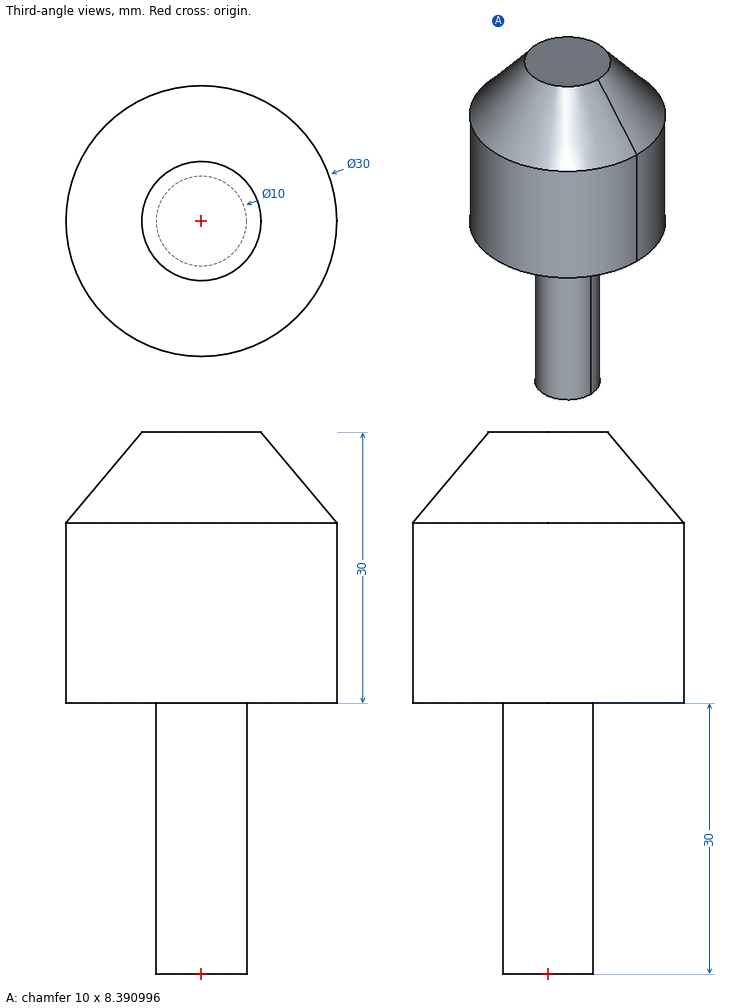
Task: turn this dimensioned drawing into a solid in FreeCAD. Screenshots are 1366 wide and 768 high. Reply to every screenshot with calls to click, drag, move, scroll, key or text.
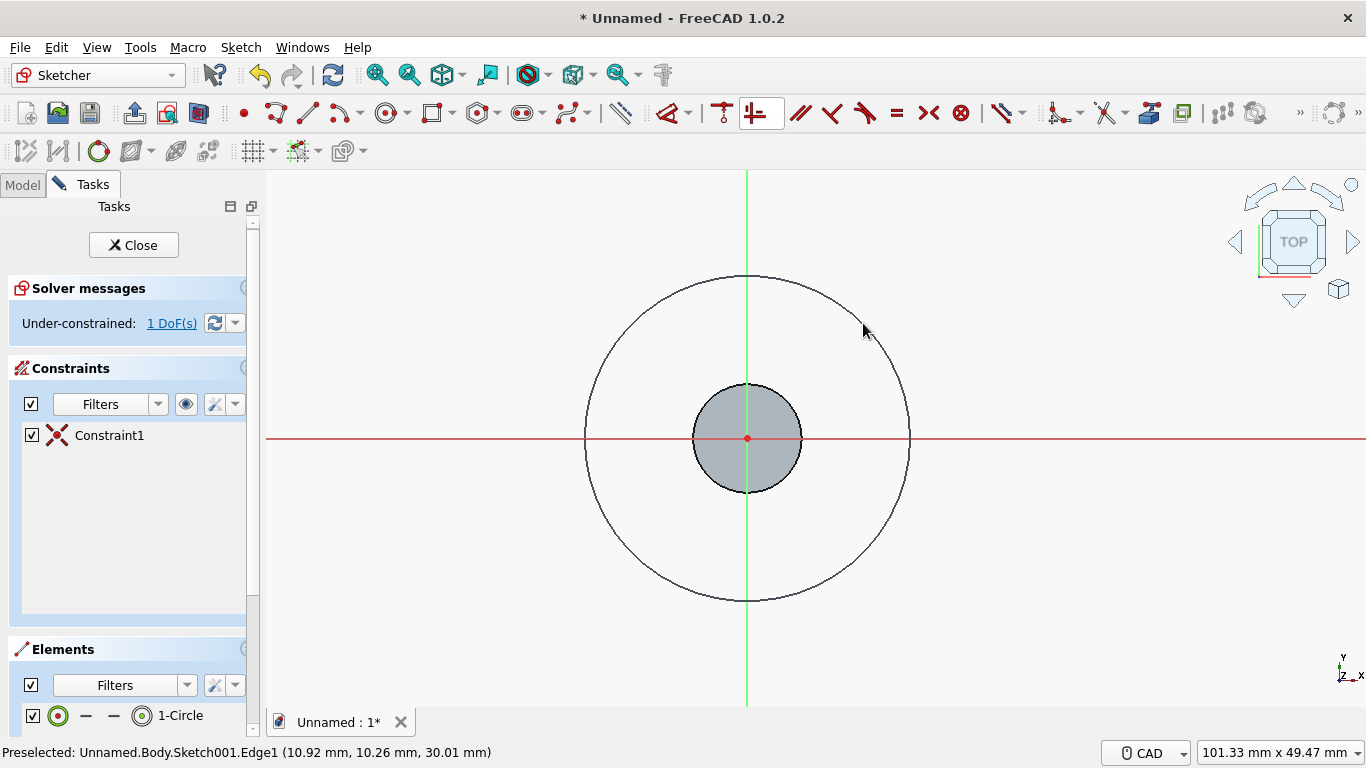
click(668, 114)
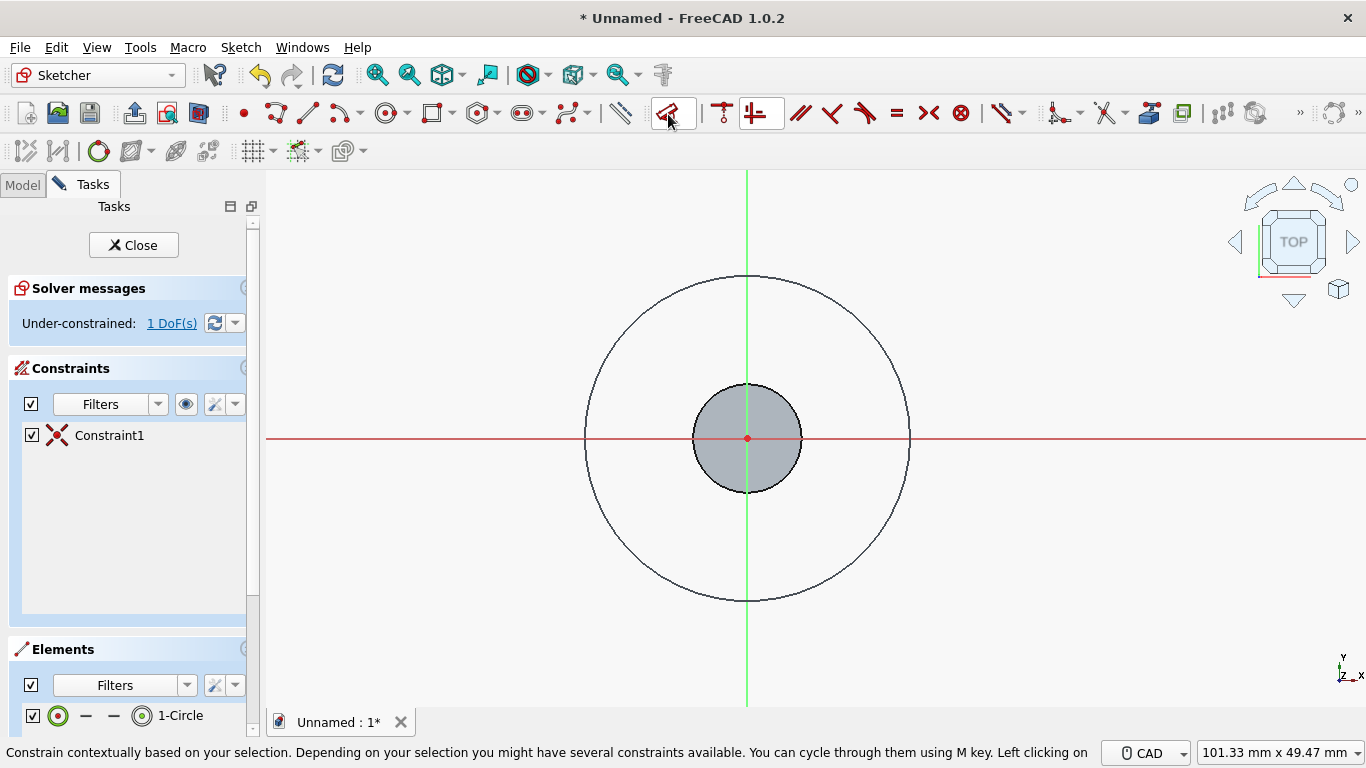
click(862, 323)
click(885, 300)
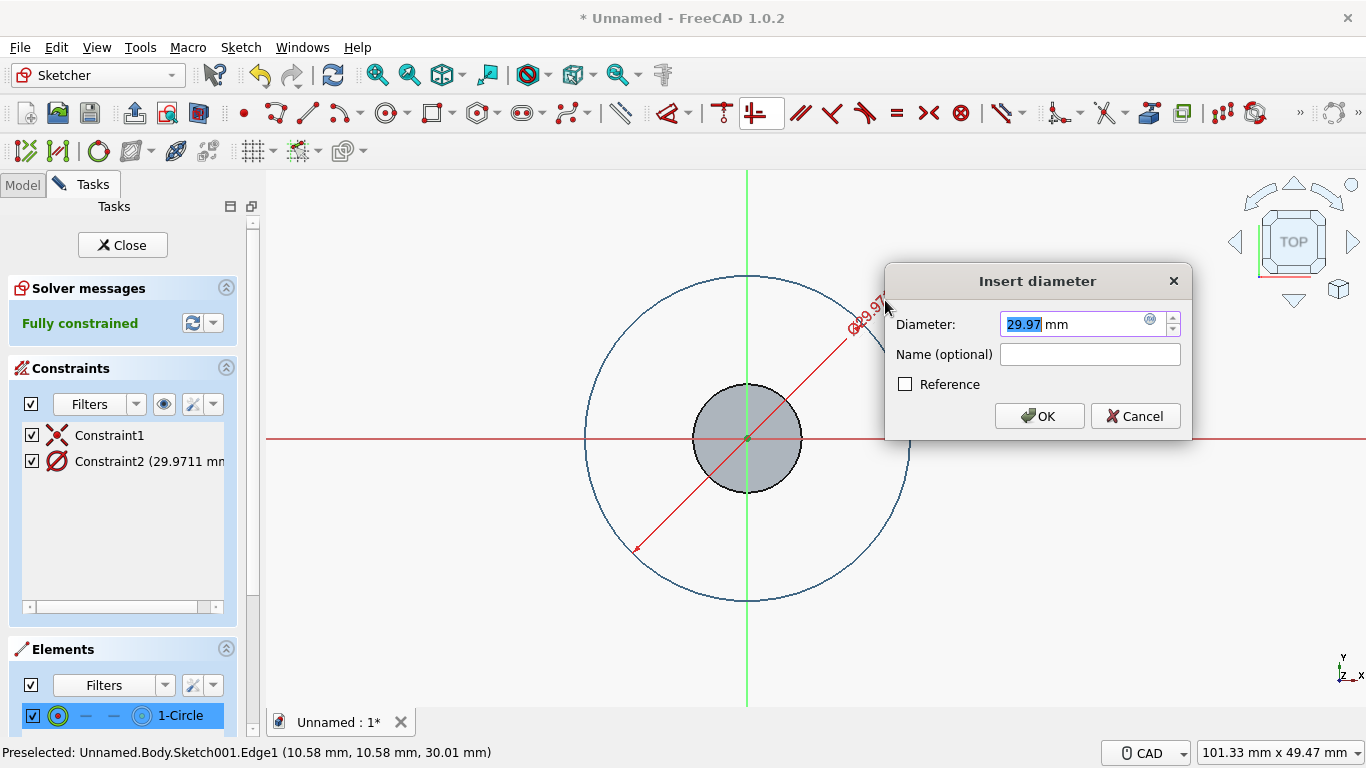
text(30)
key(Return)
key(Escape)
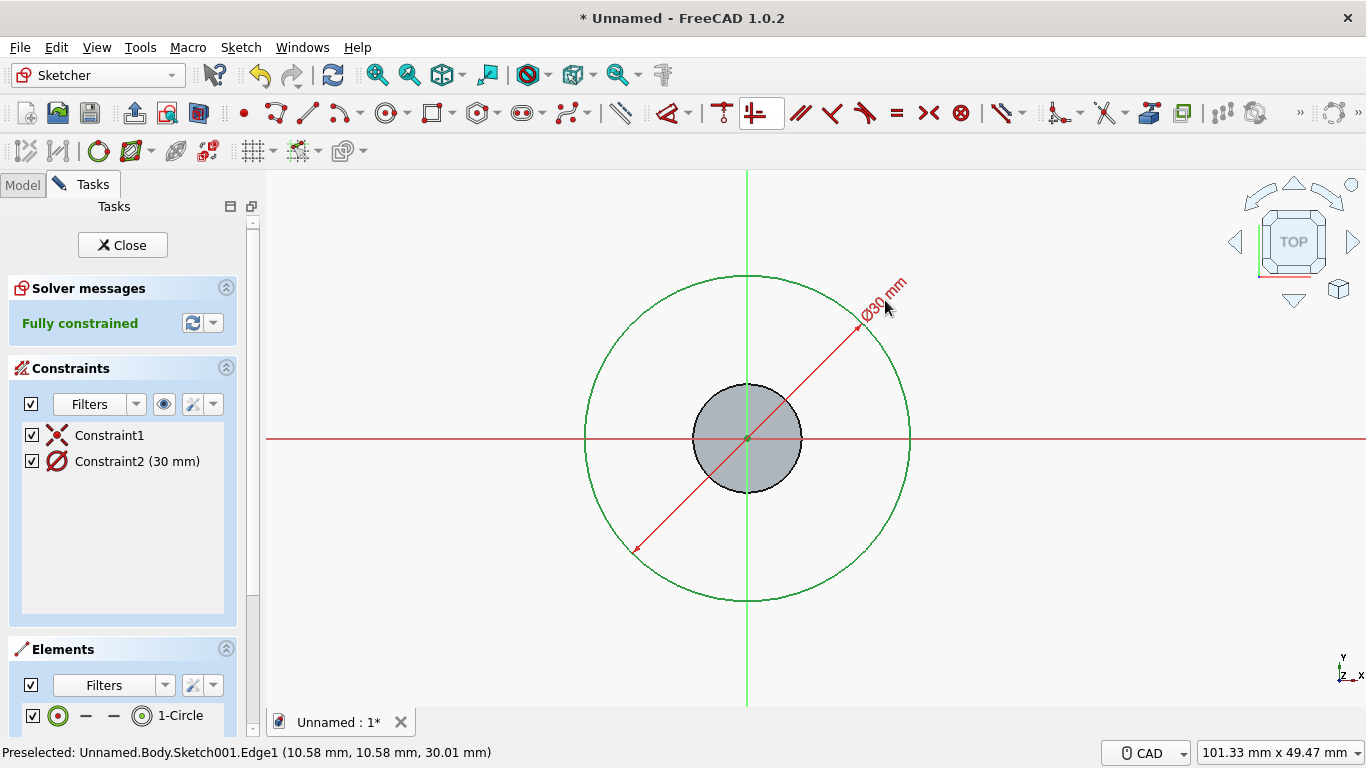
click(123, 245)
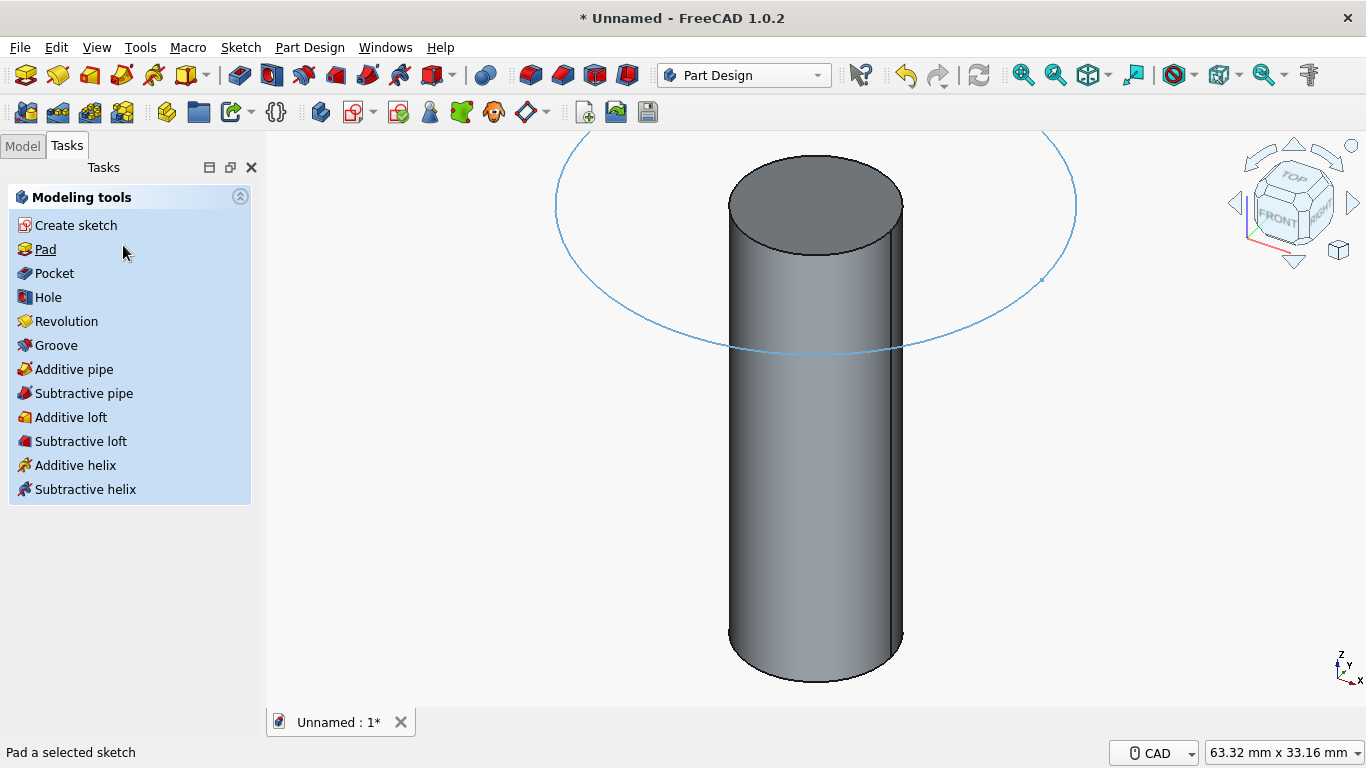
click(26, 76)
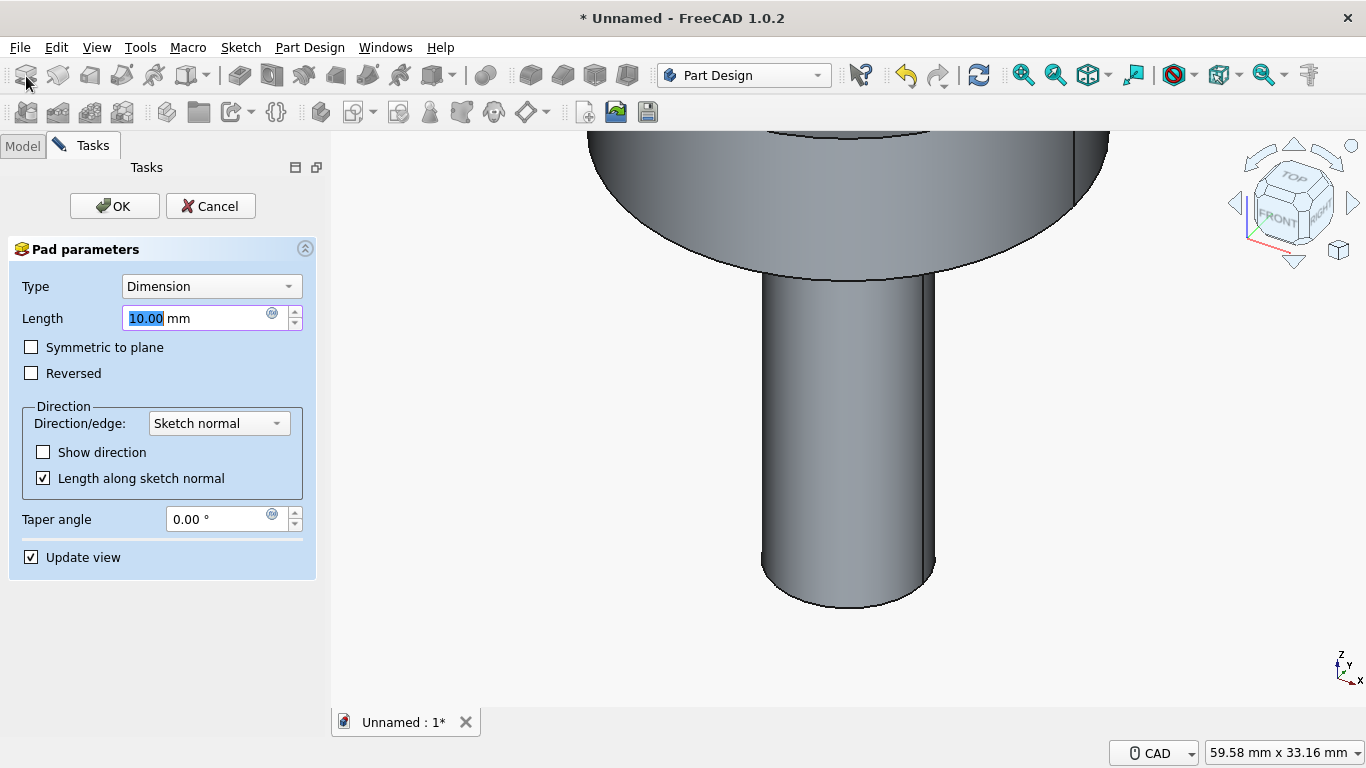
text(30)
key(Tab)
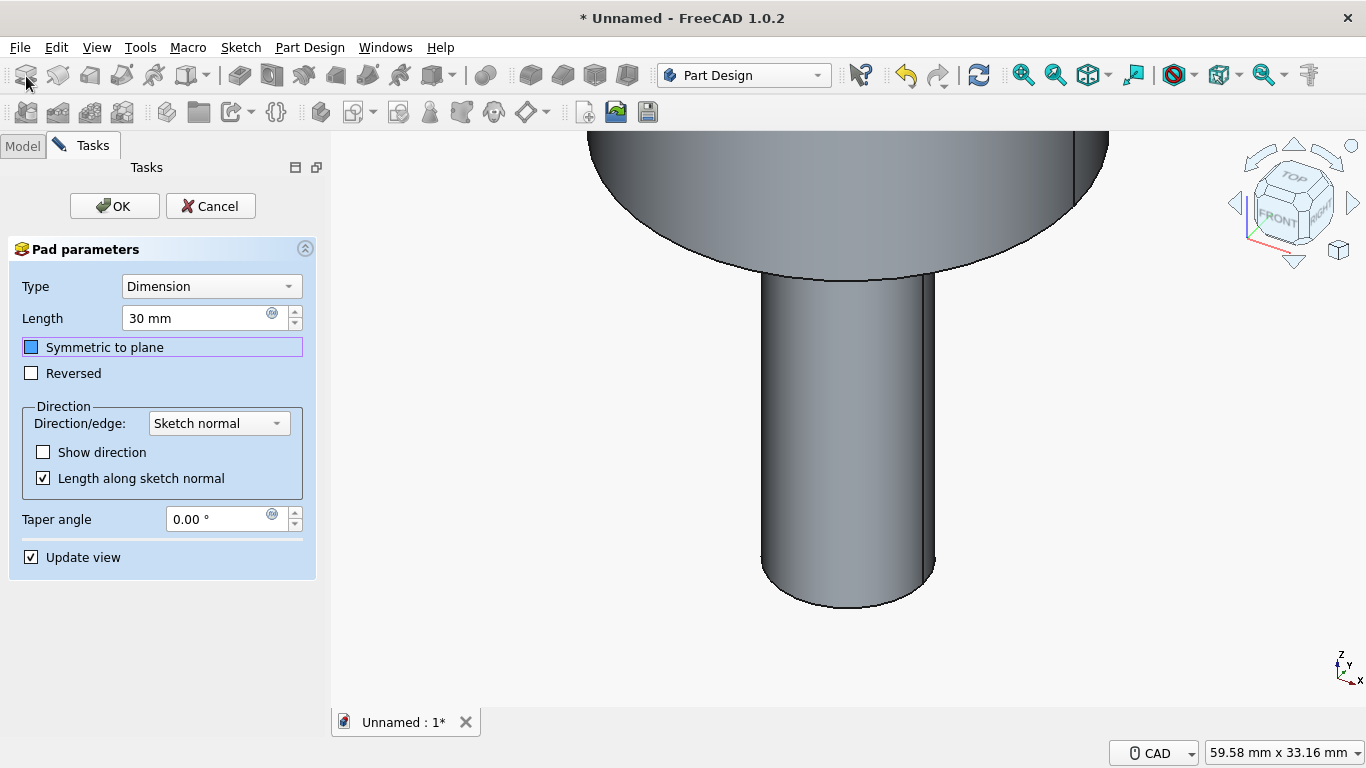
click(115, 206)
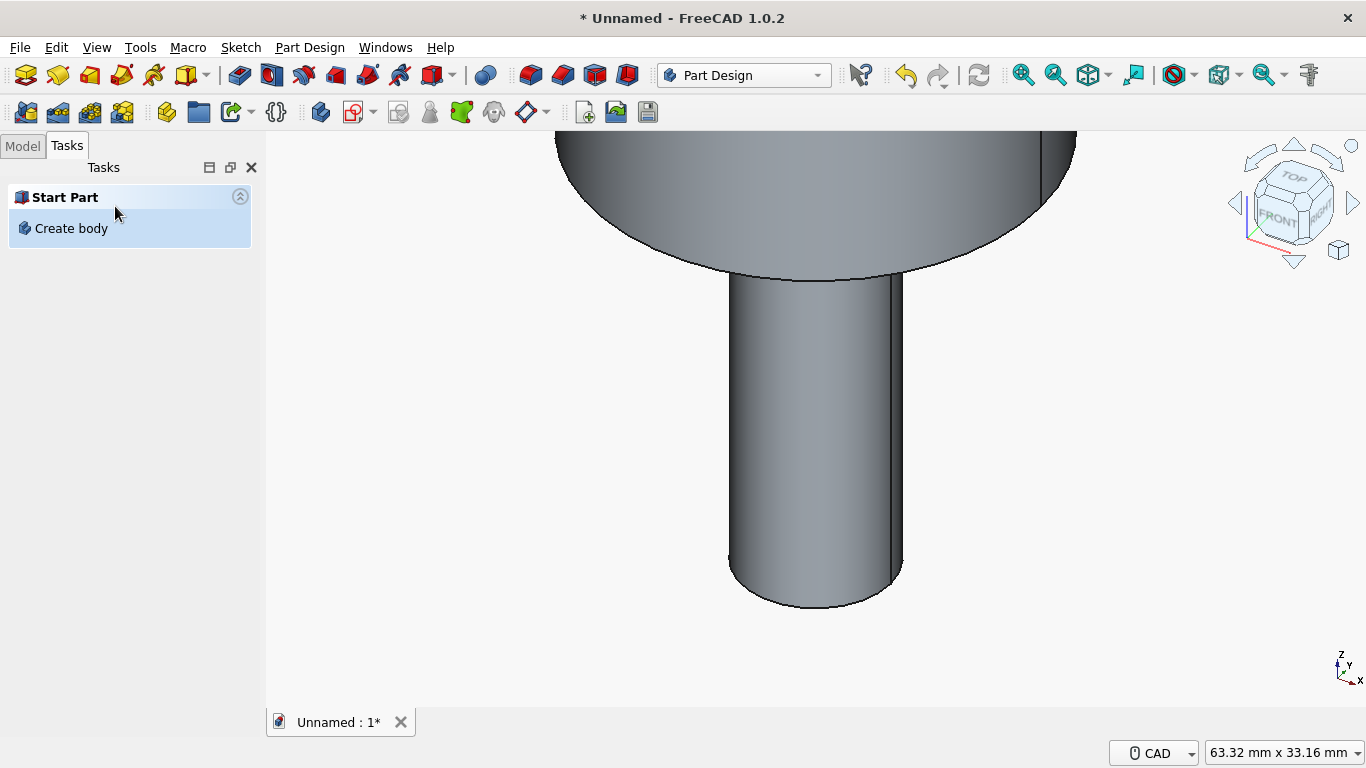
click(1024, 76)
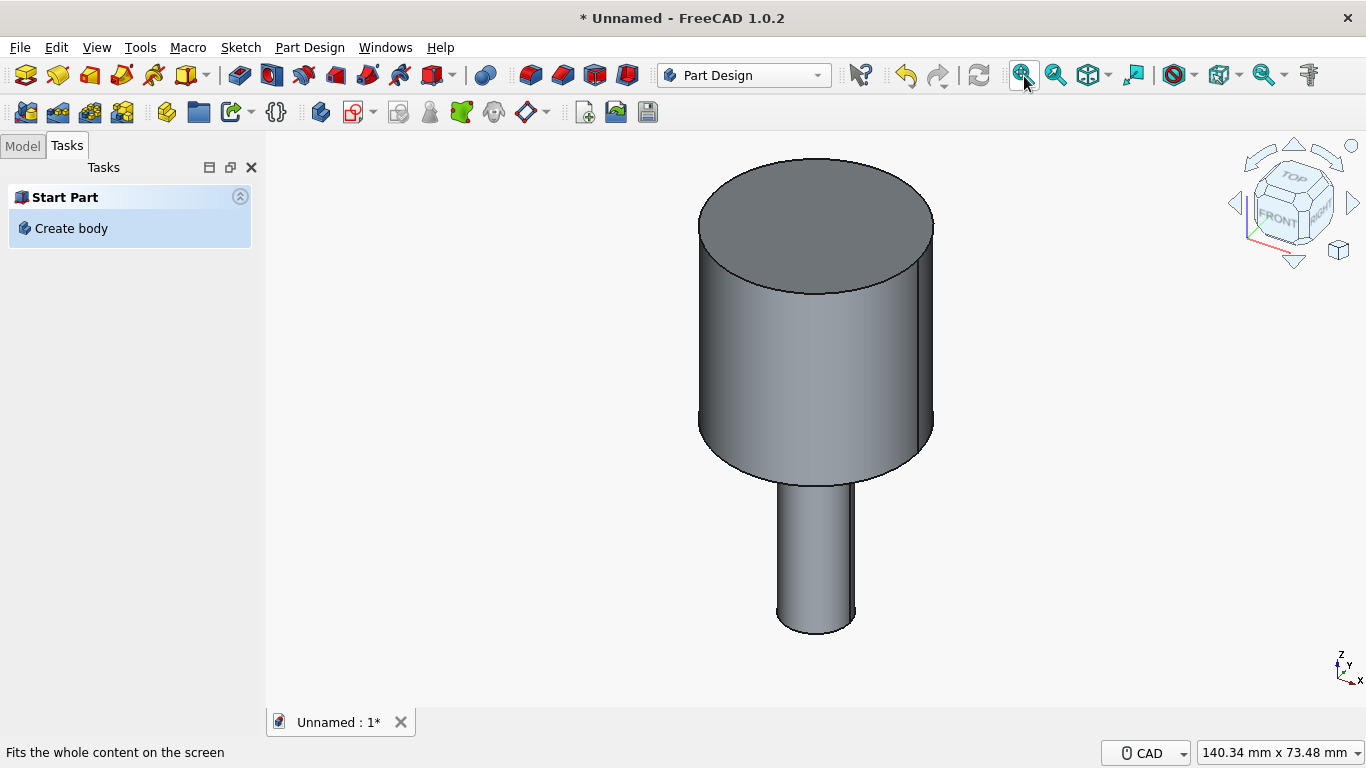
click(699, 232)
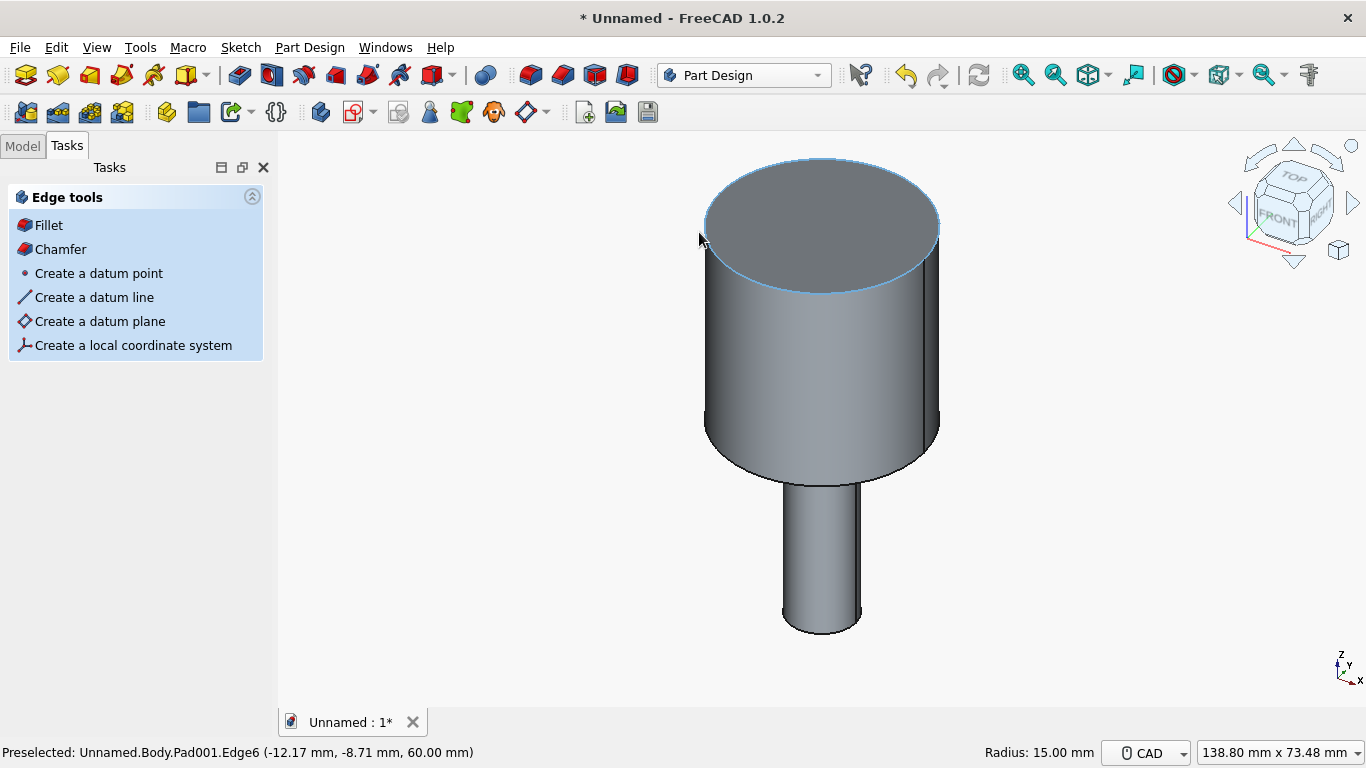
click(564, 76)